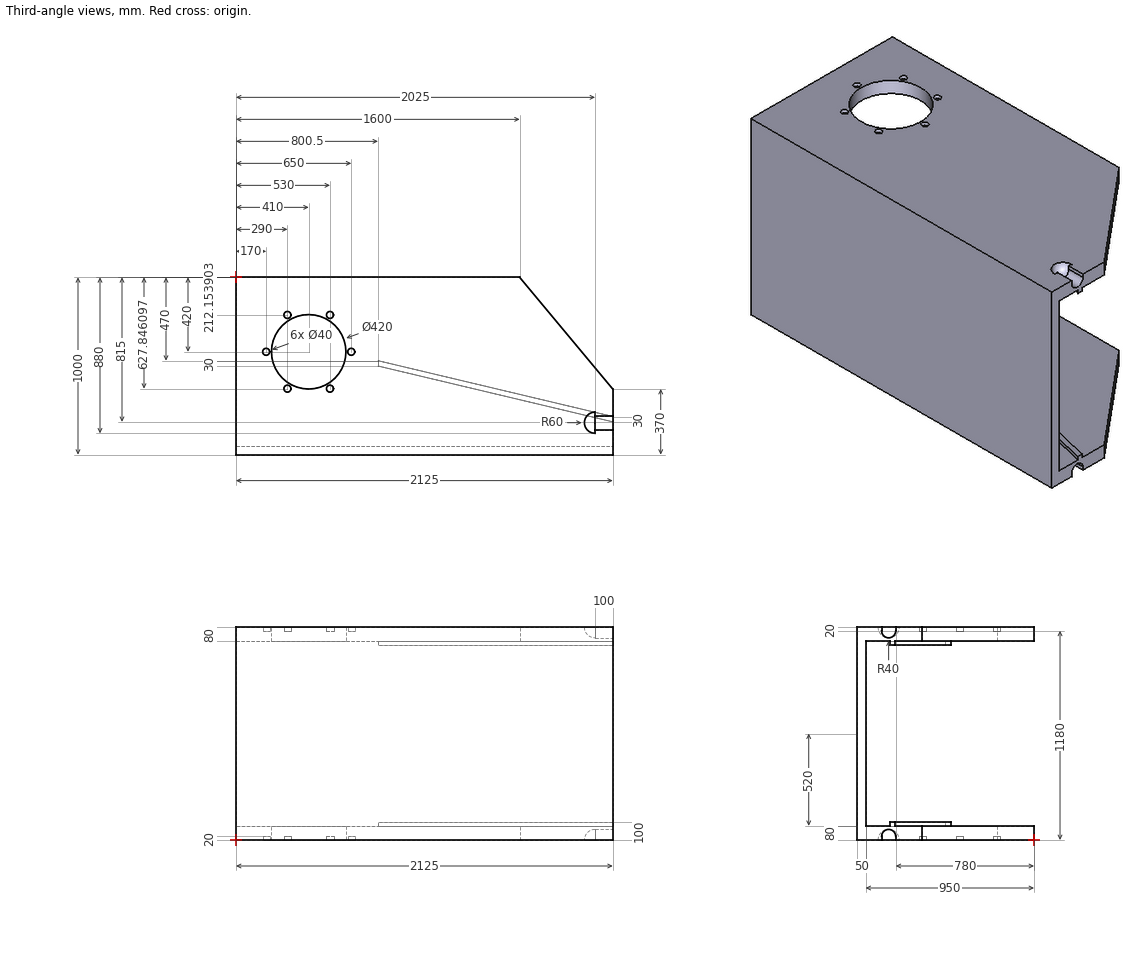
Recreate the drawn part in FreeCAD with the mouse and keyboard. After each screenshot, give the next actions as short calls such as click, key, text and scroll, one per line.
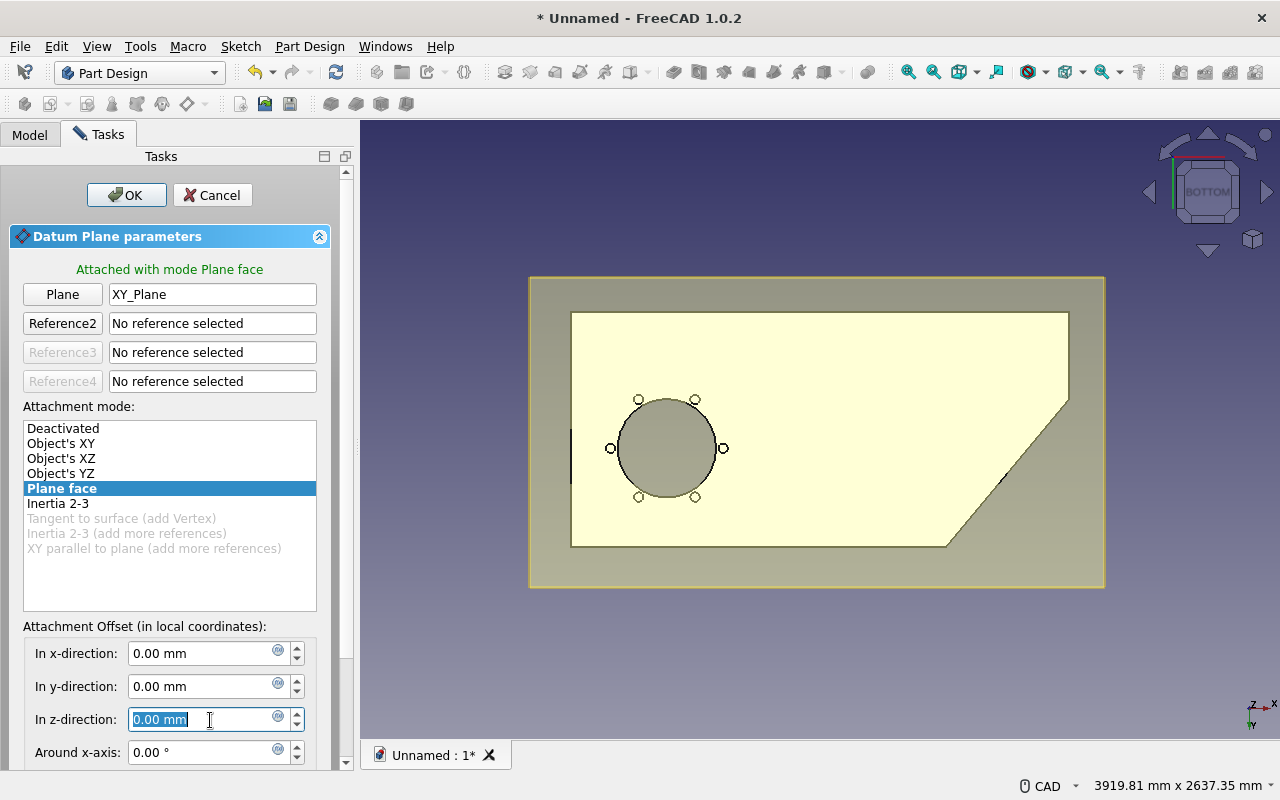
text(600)
key(Tab)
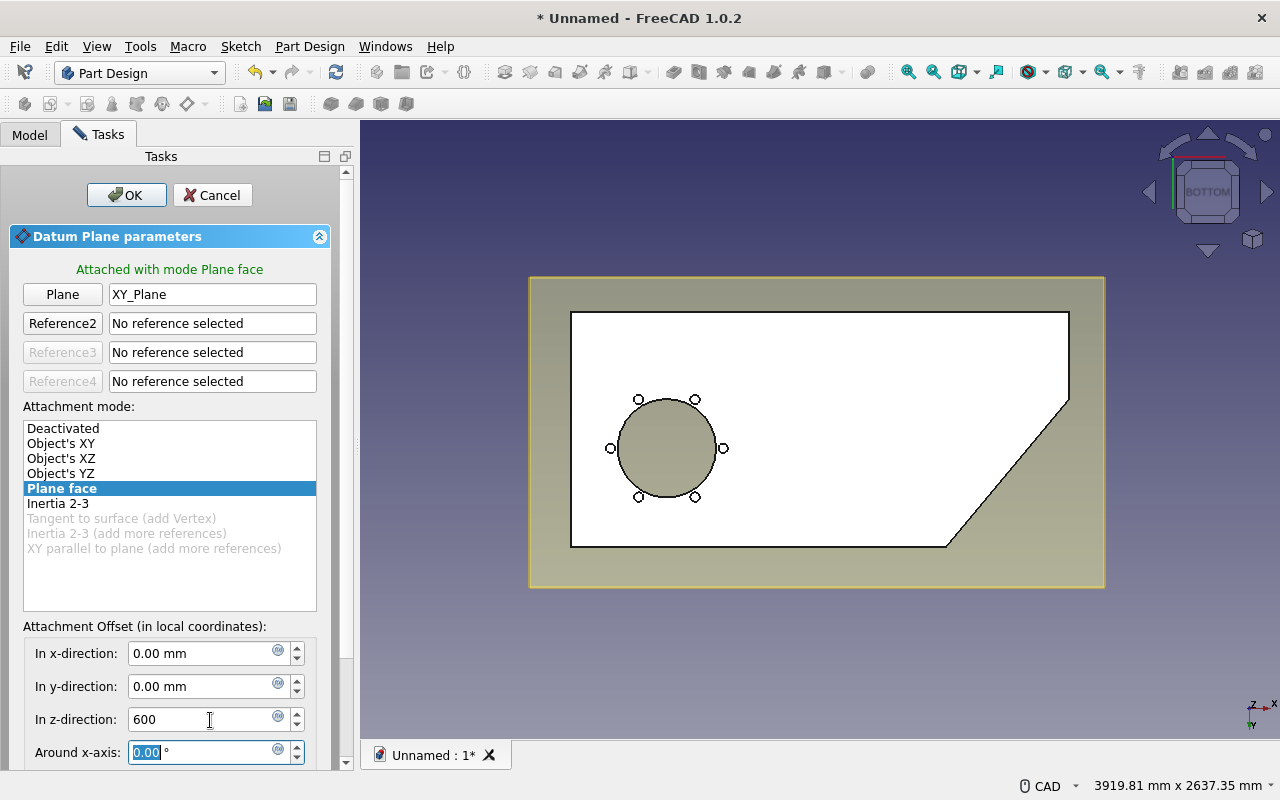
click(127, 195)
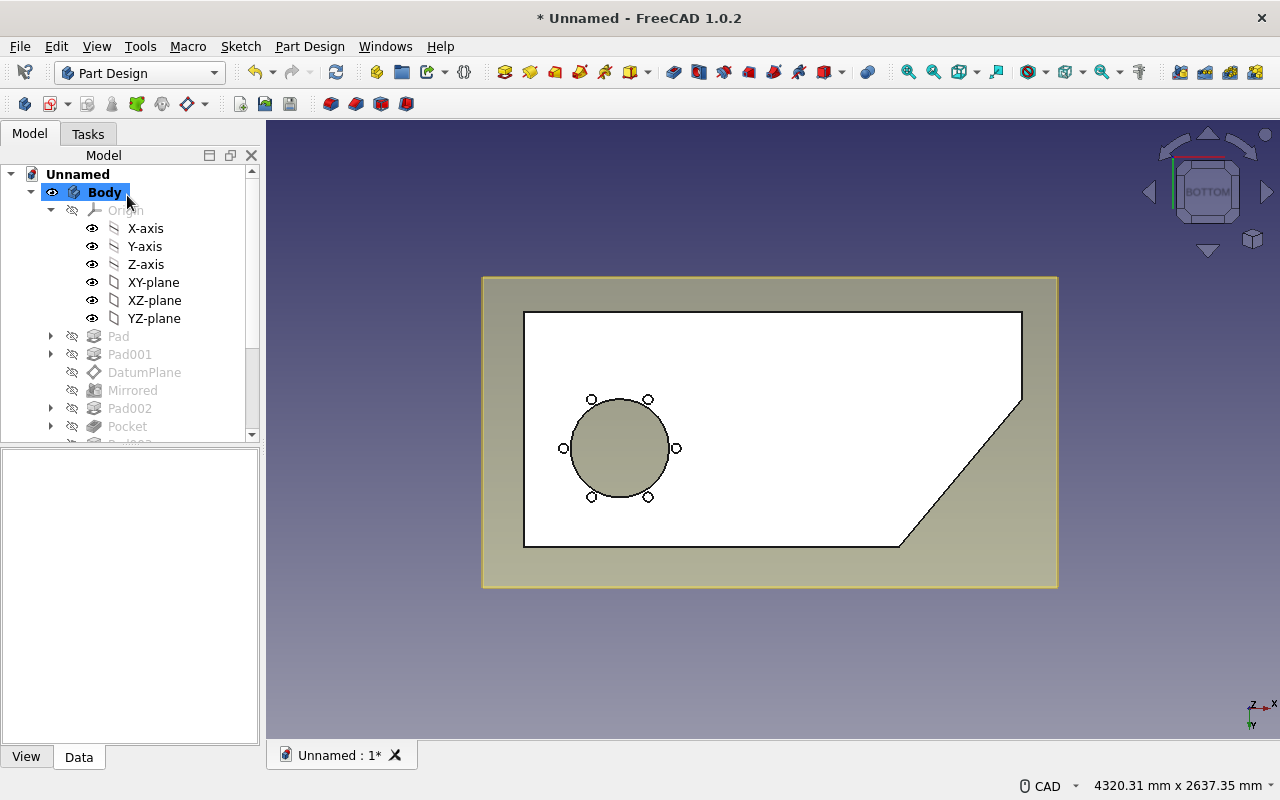
scroll(101, 296, down, 3)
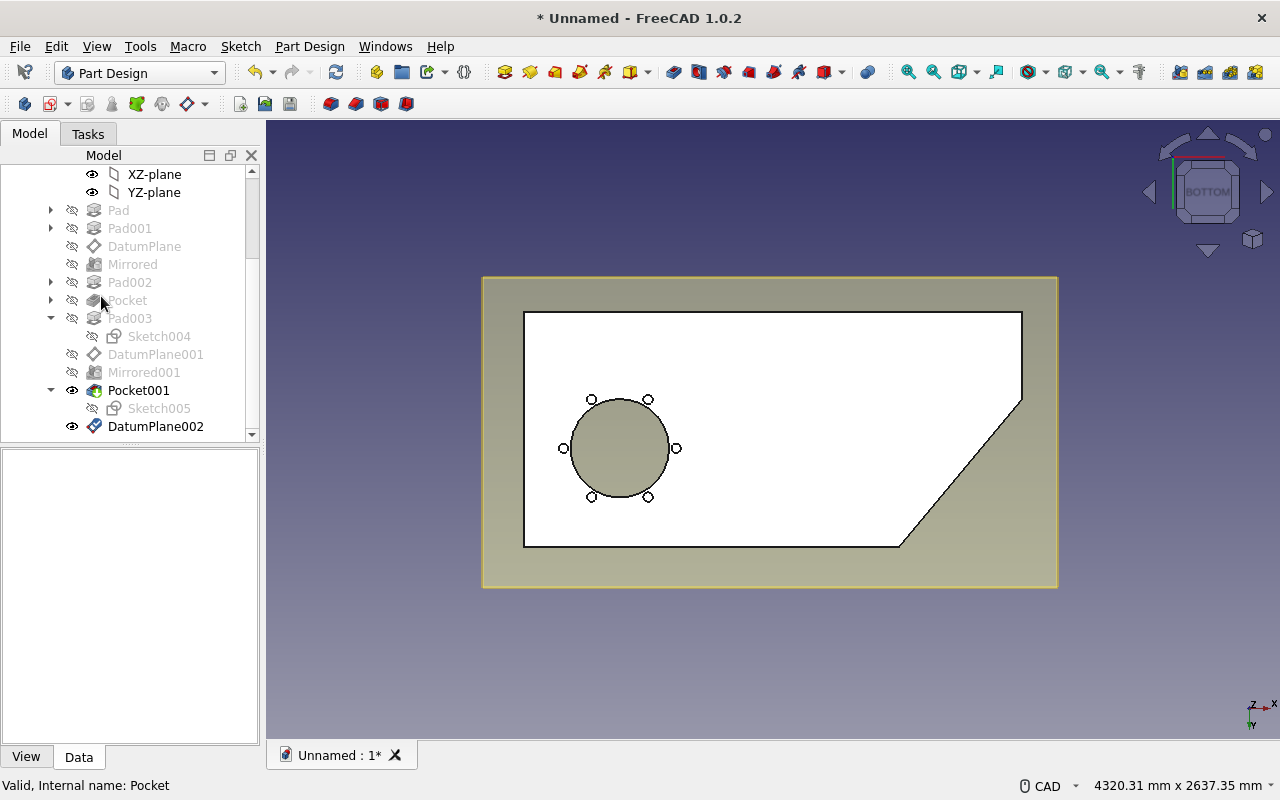
click(117, 390)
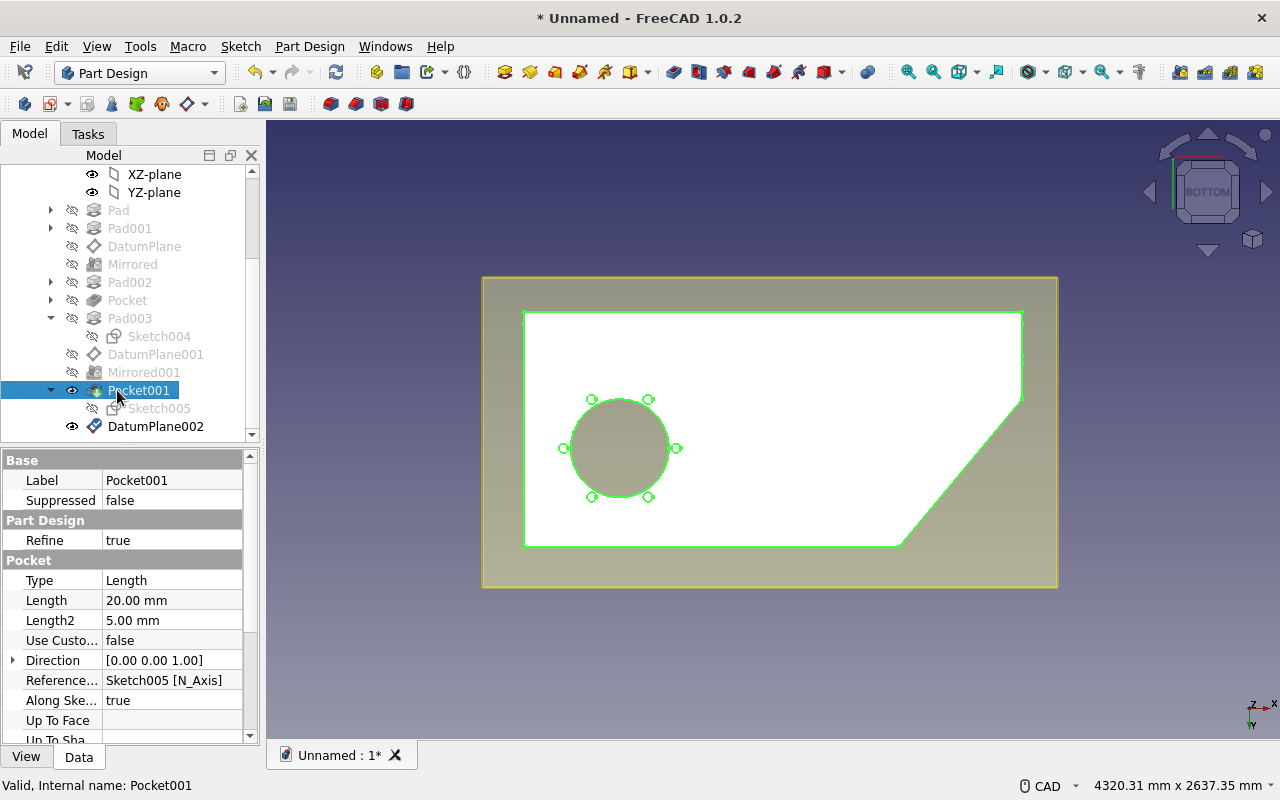
click(1180, 72)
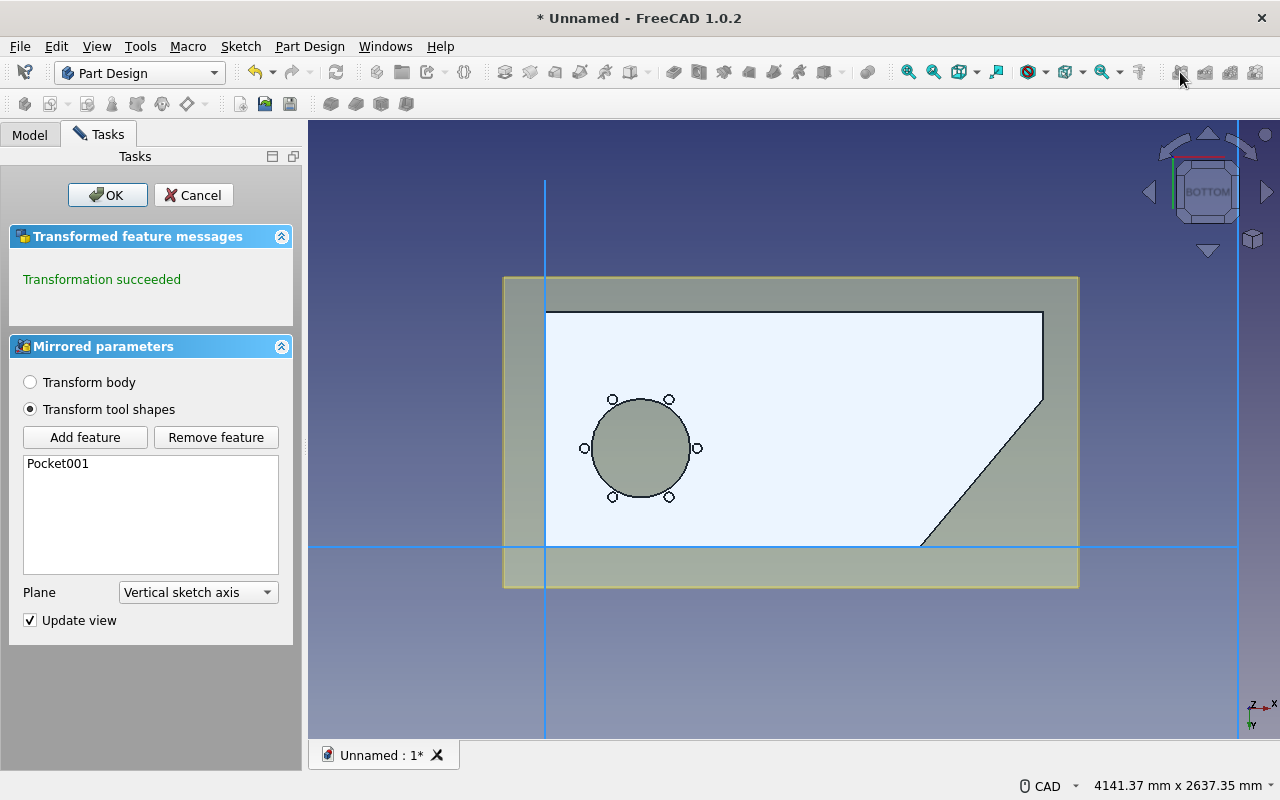
click(199, 592)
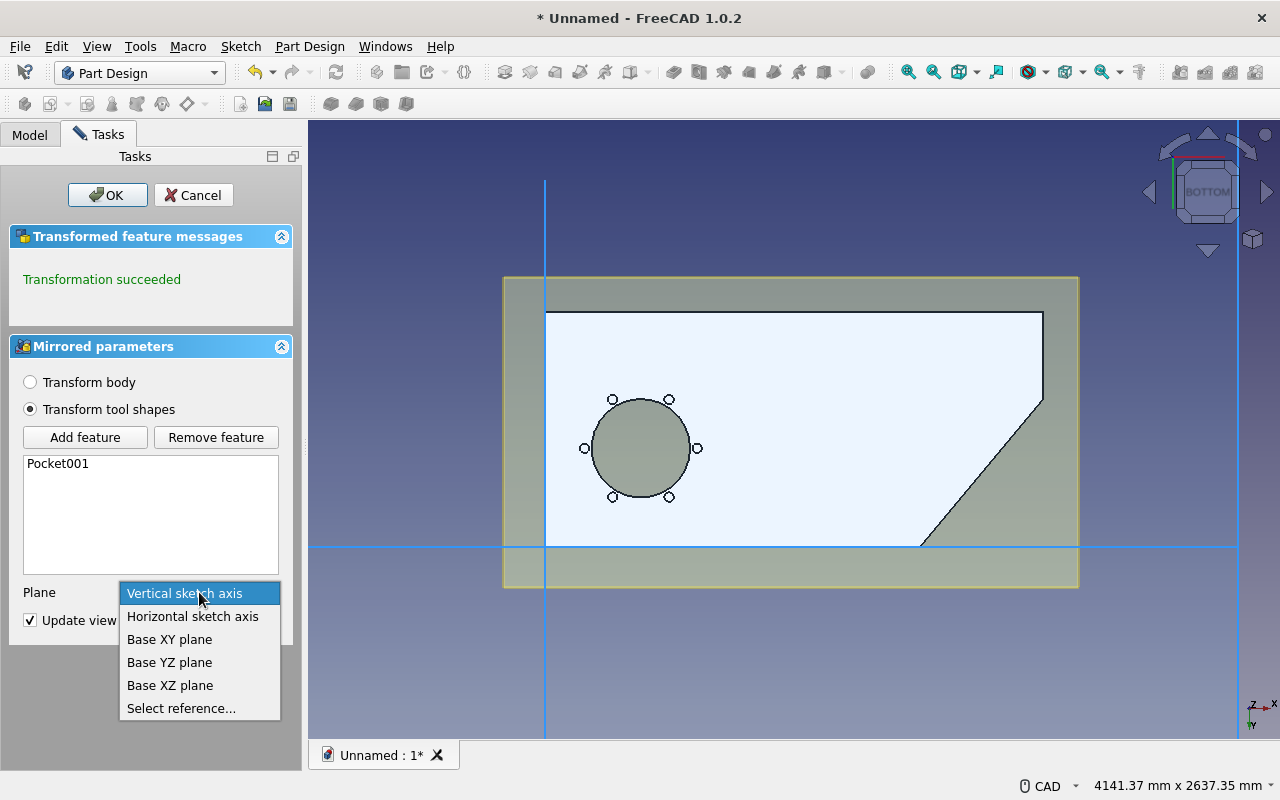
click(198, 708)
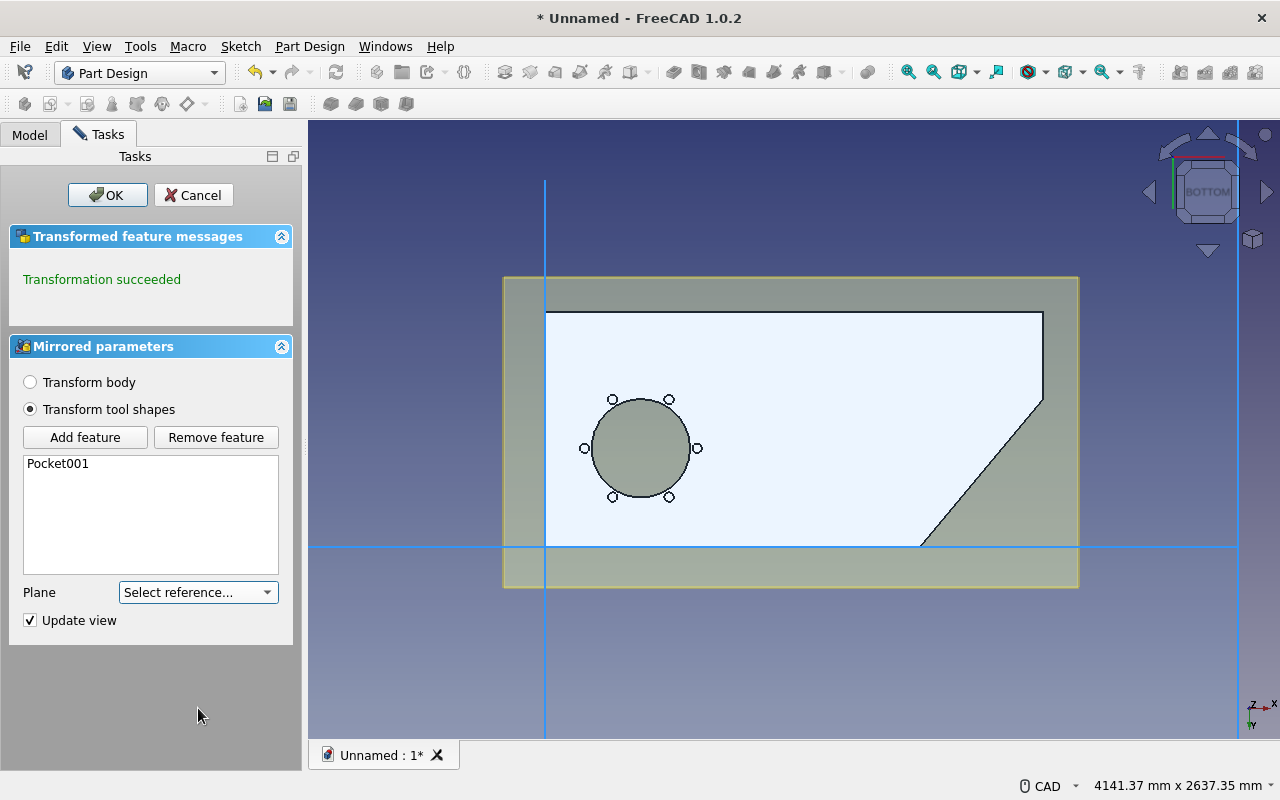
click(30, 134)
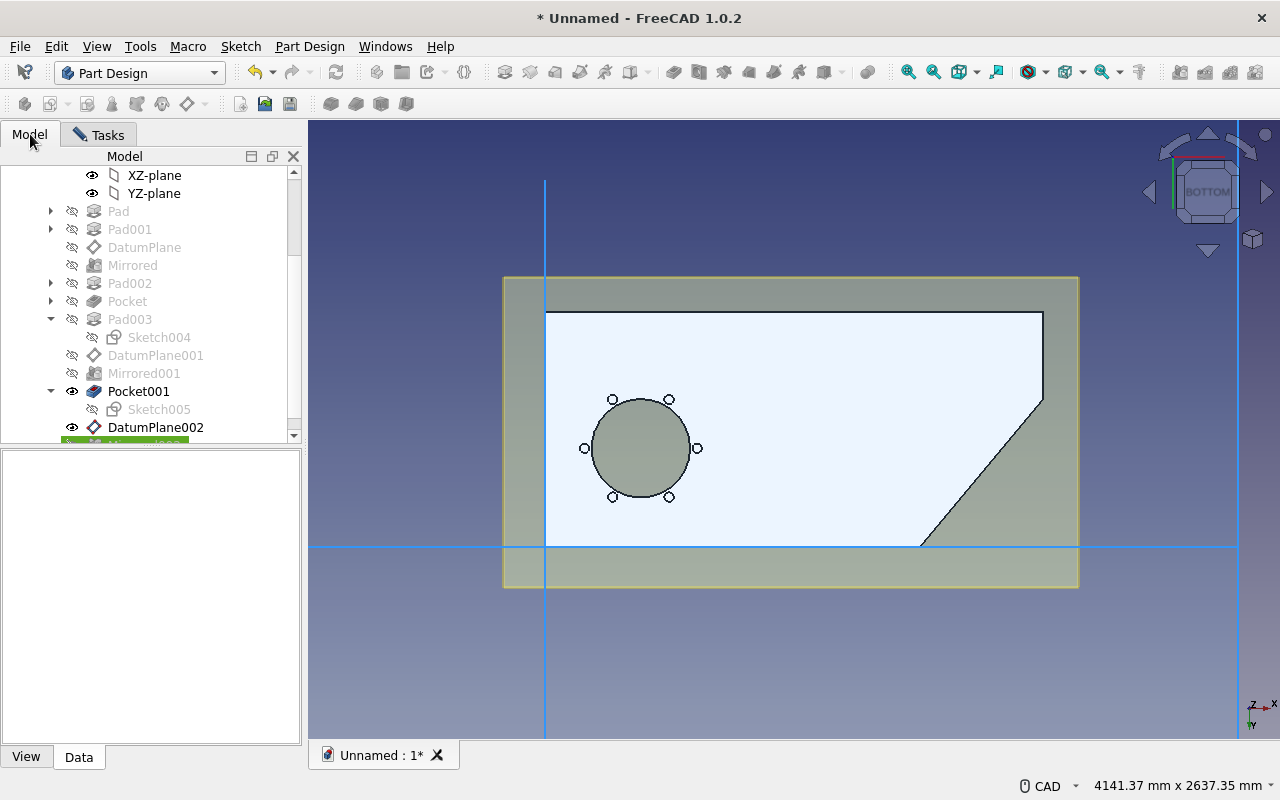
click(117, 427)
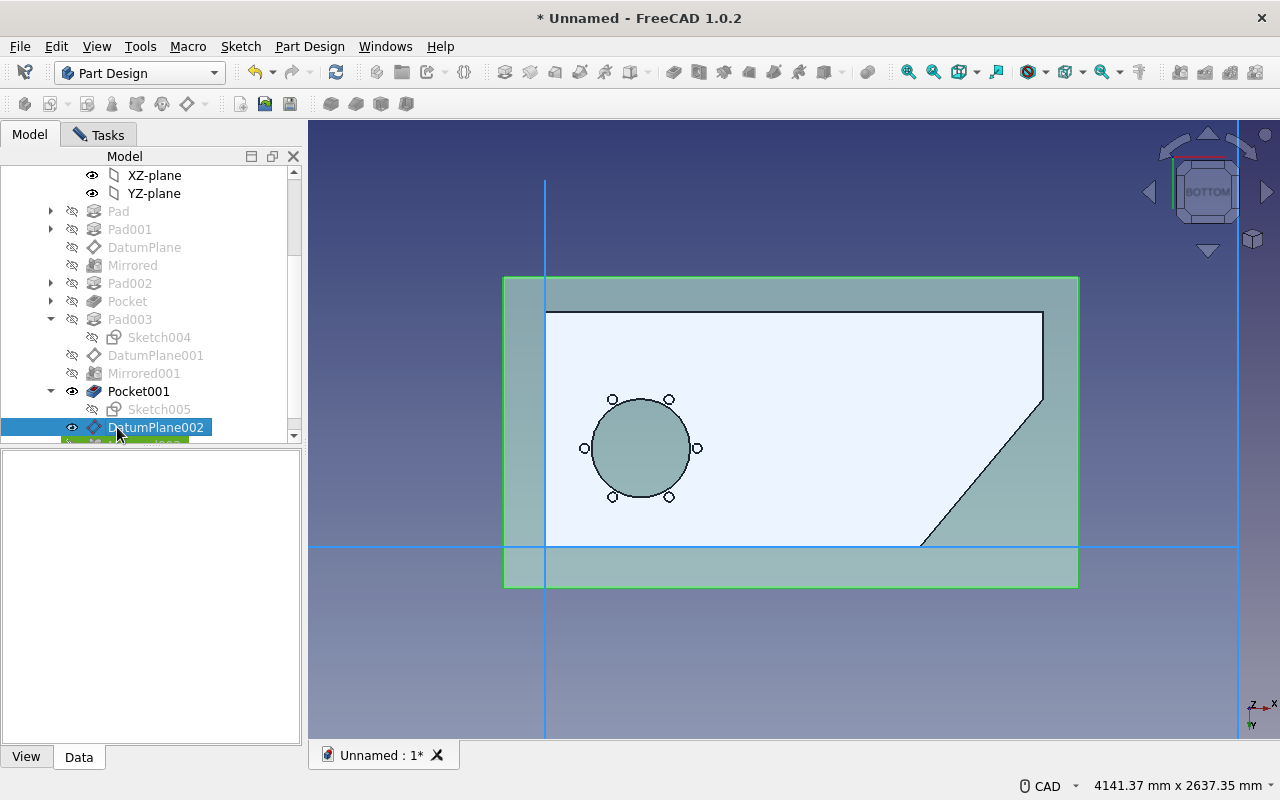
click(98, 134)